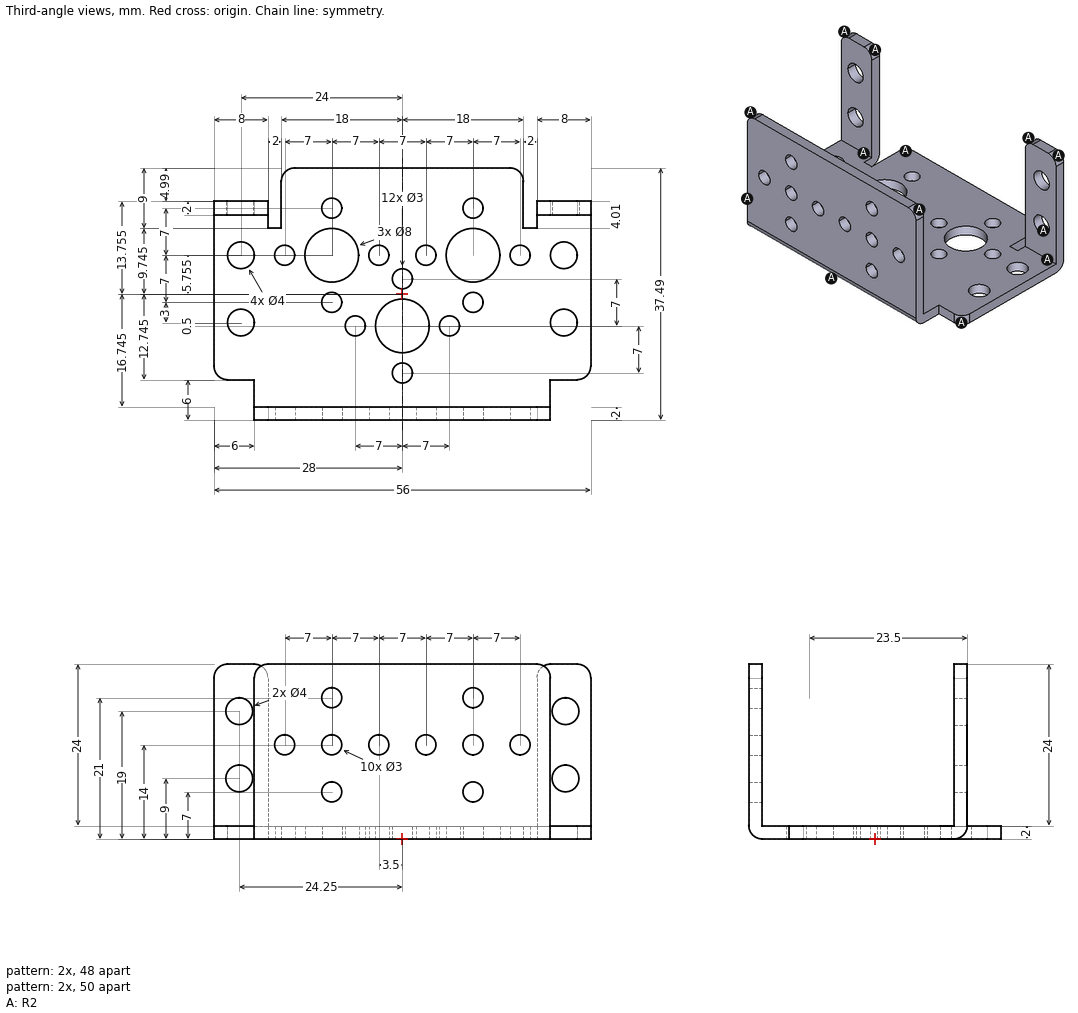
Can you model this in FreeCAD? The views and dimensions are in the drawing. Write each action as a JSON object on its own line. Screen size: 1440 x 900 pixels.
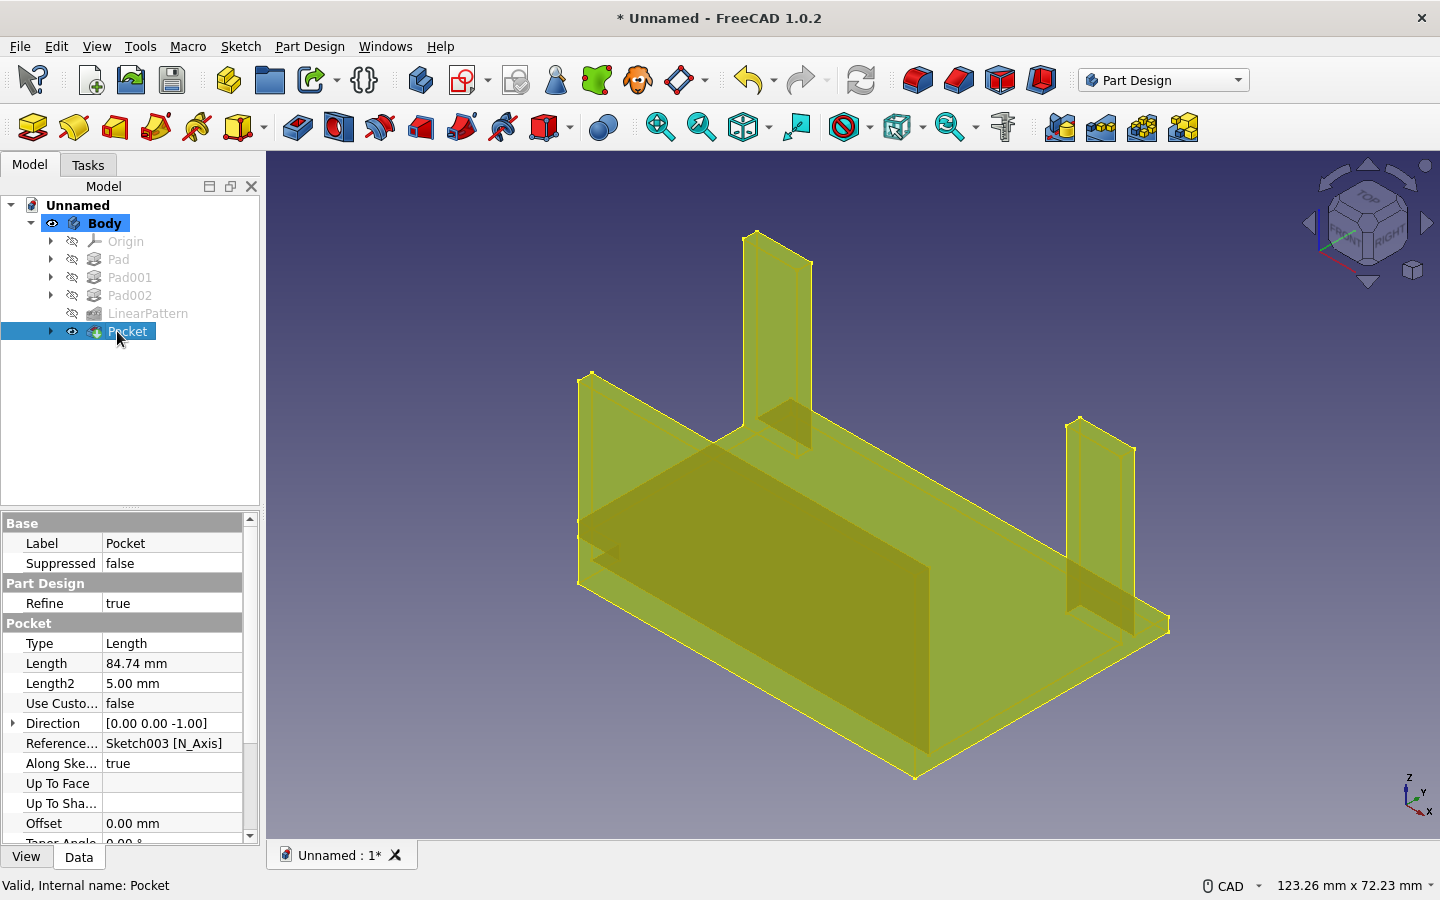
{"action": "left_click", "coordinate": [1101, 128]}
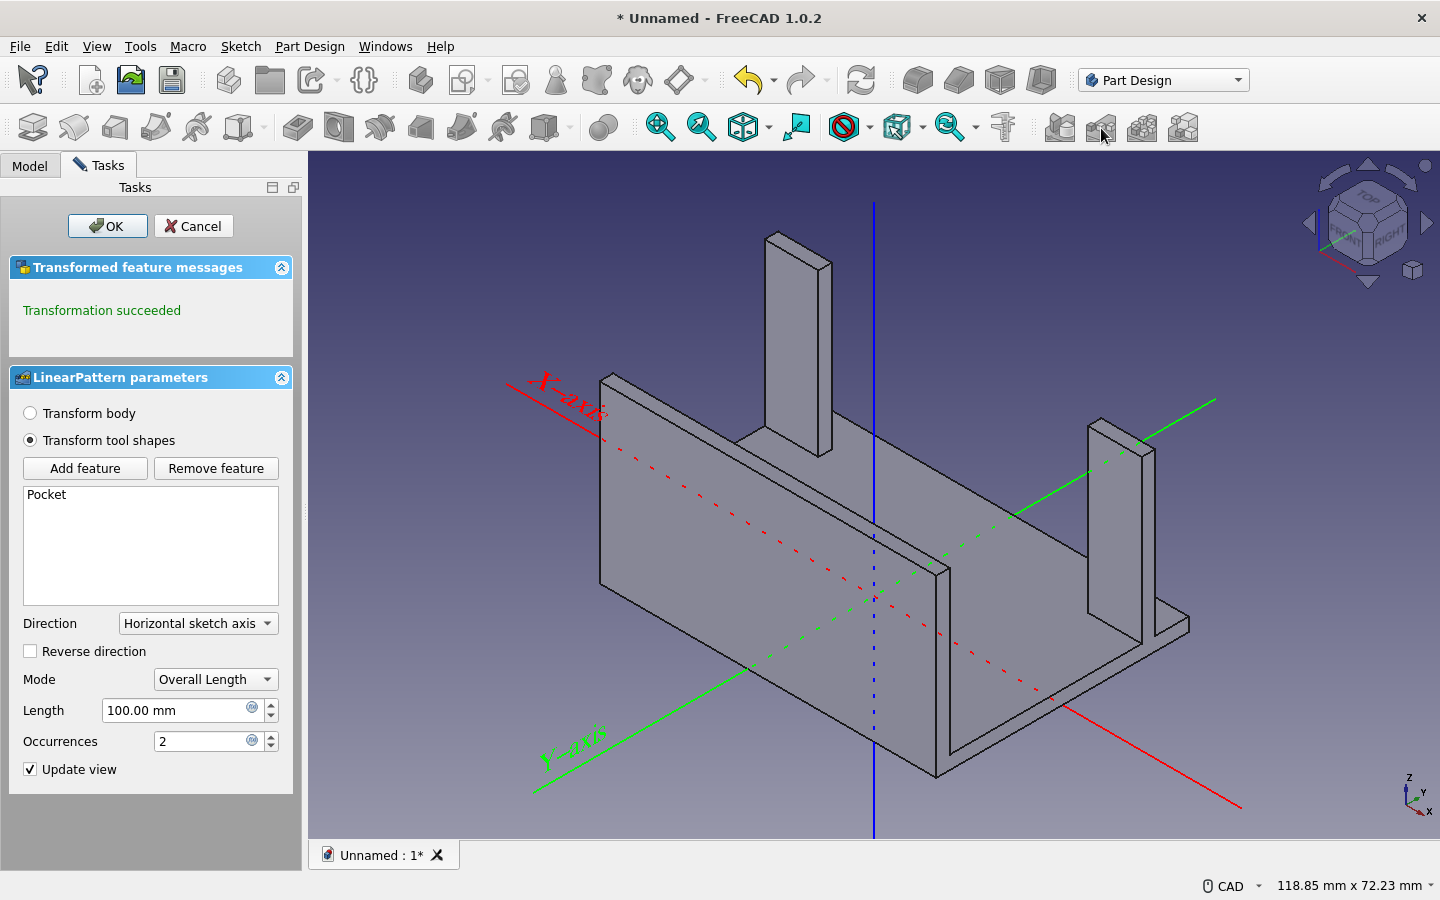
{"action": "left_click", "coordinate": [199, 624]}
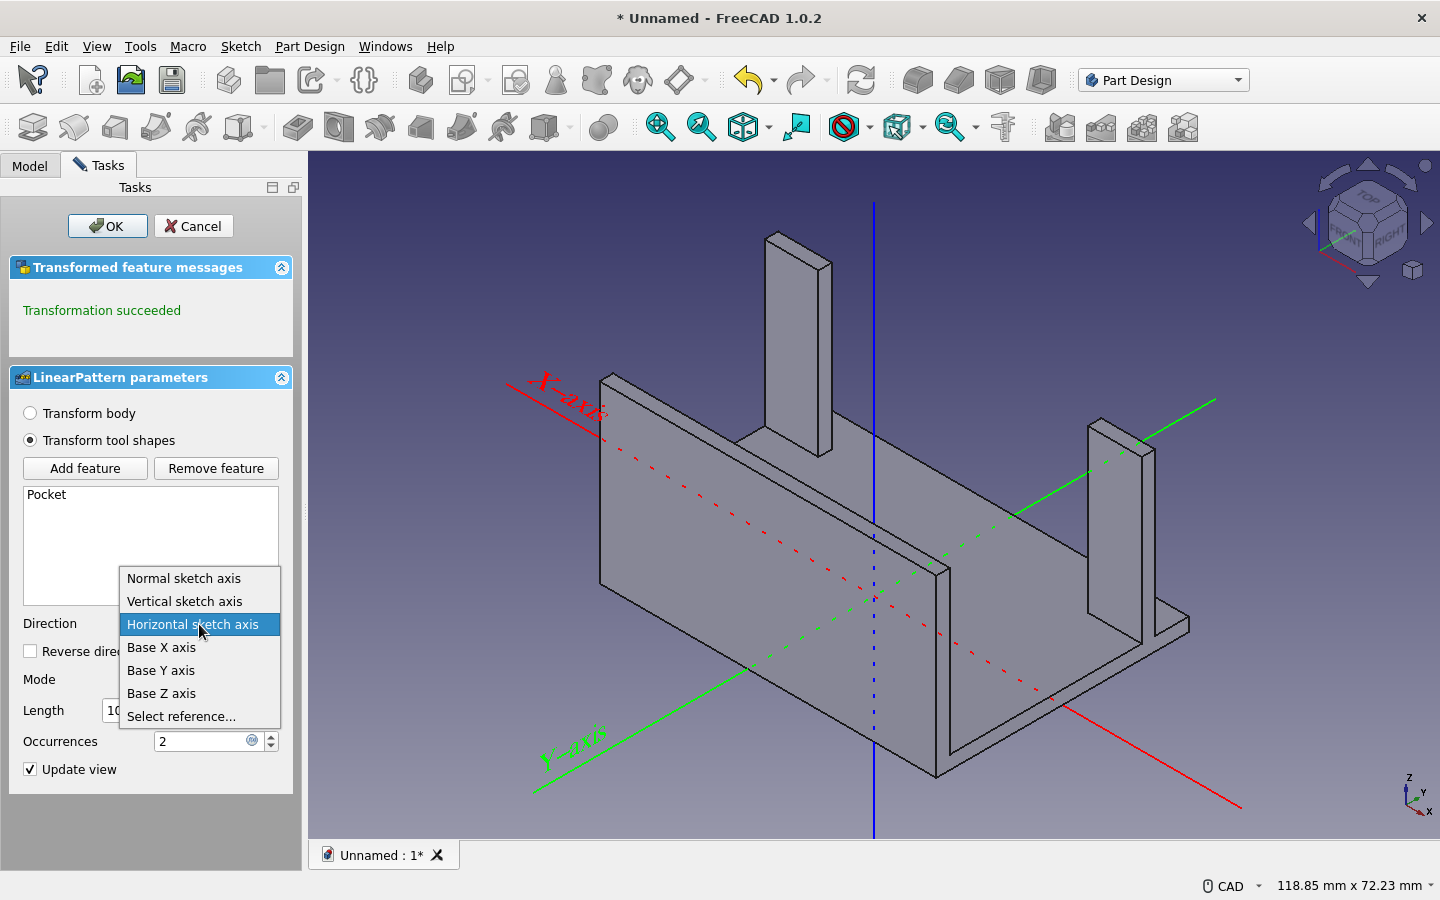
{"action": "left_click", "coordinate": [198, 648]}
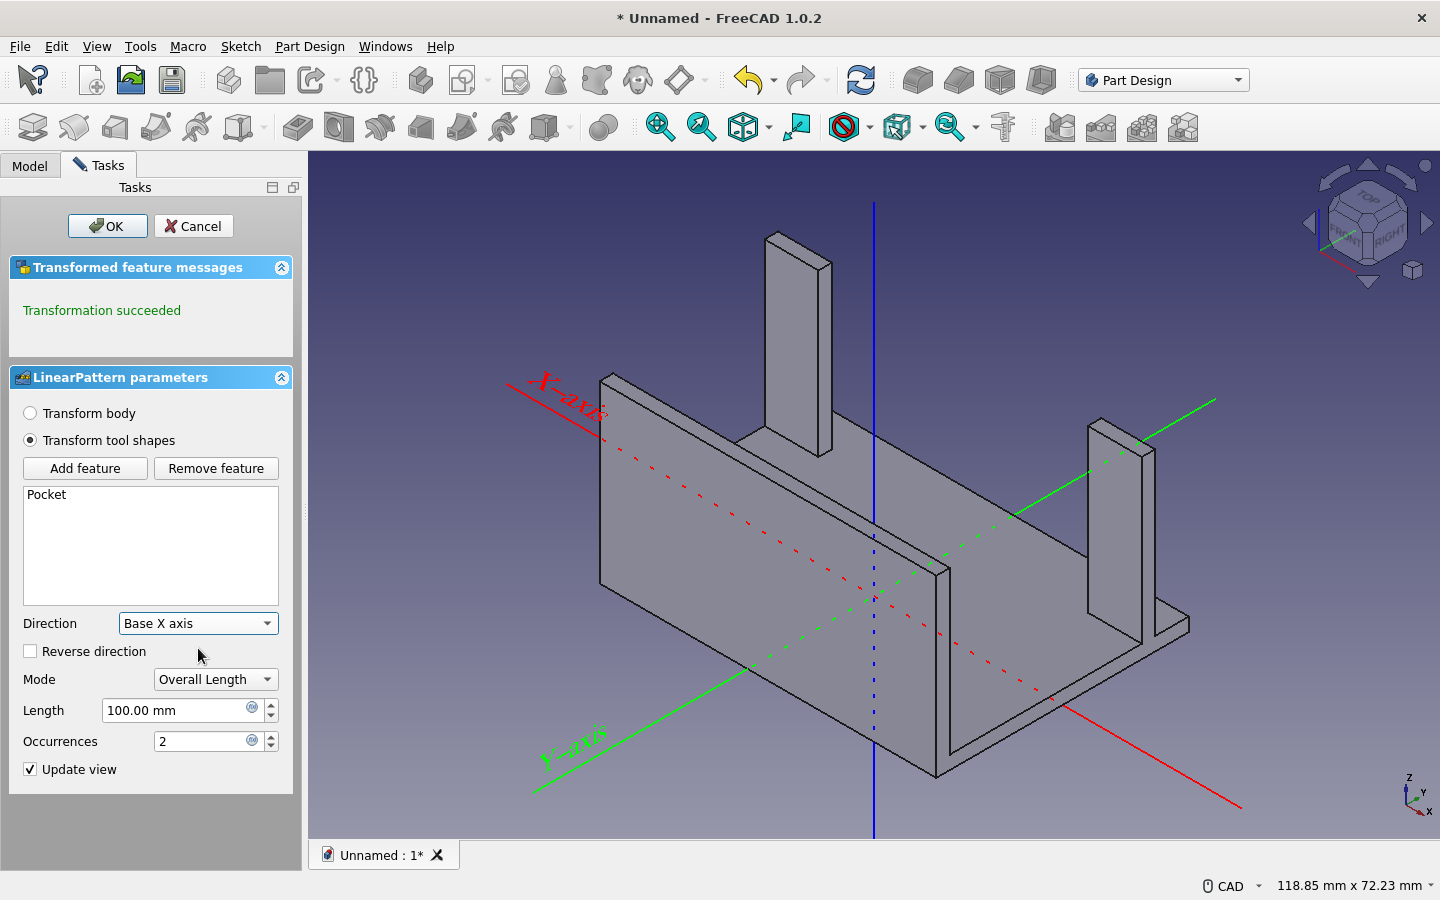
{"action": "left_click", "coordinate": [216, 680]}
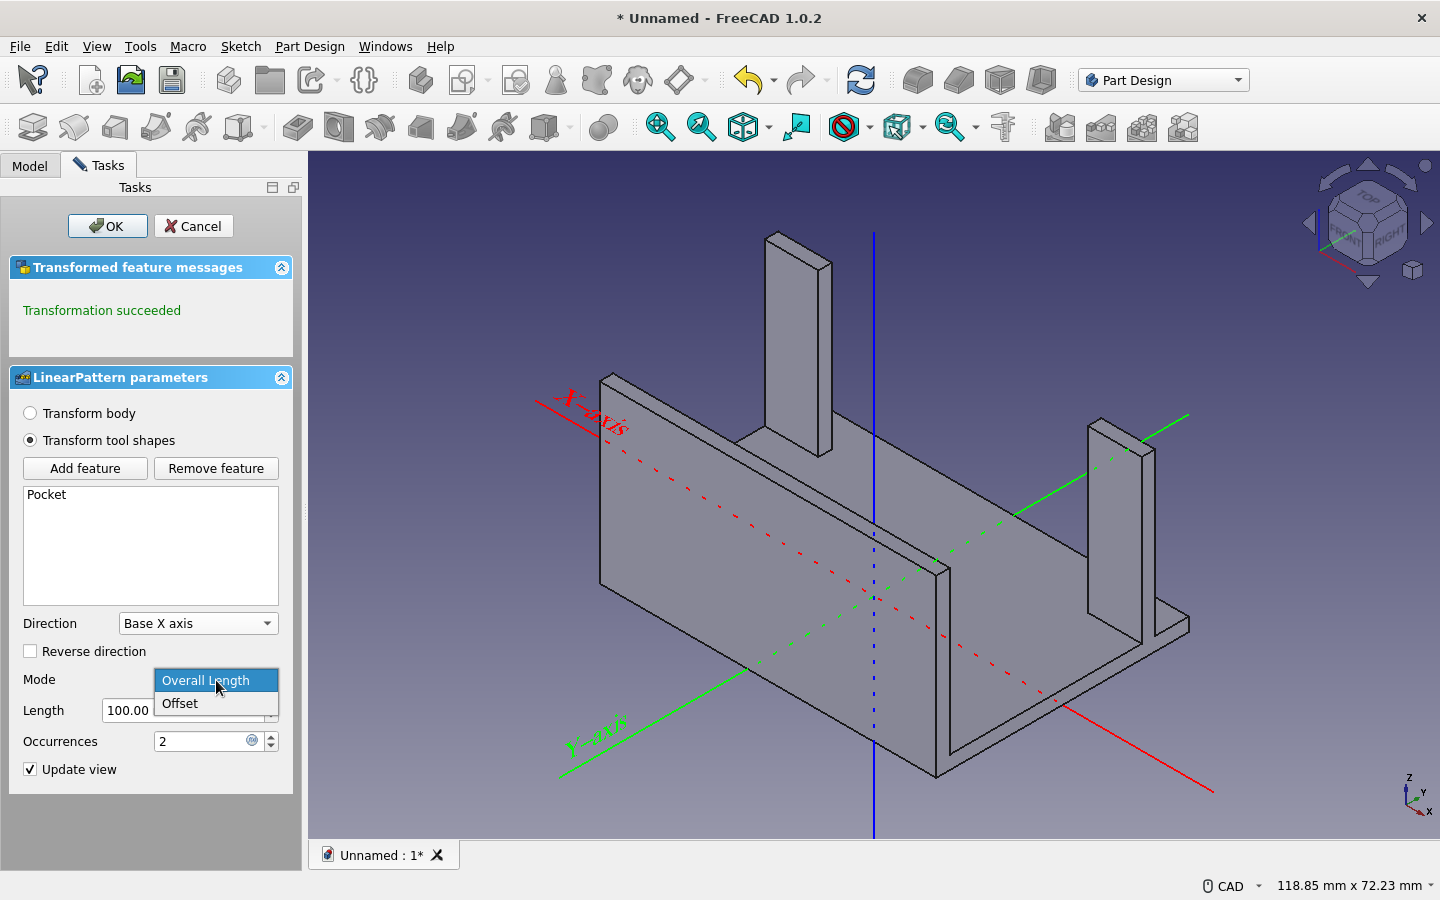
{"action": "left_click", "coordinate": [214, 704]}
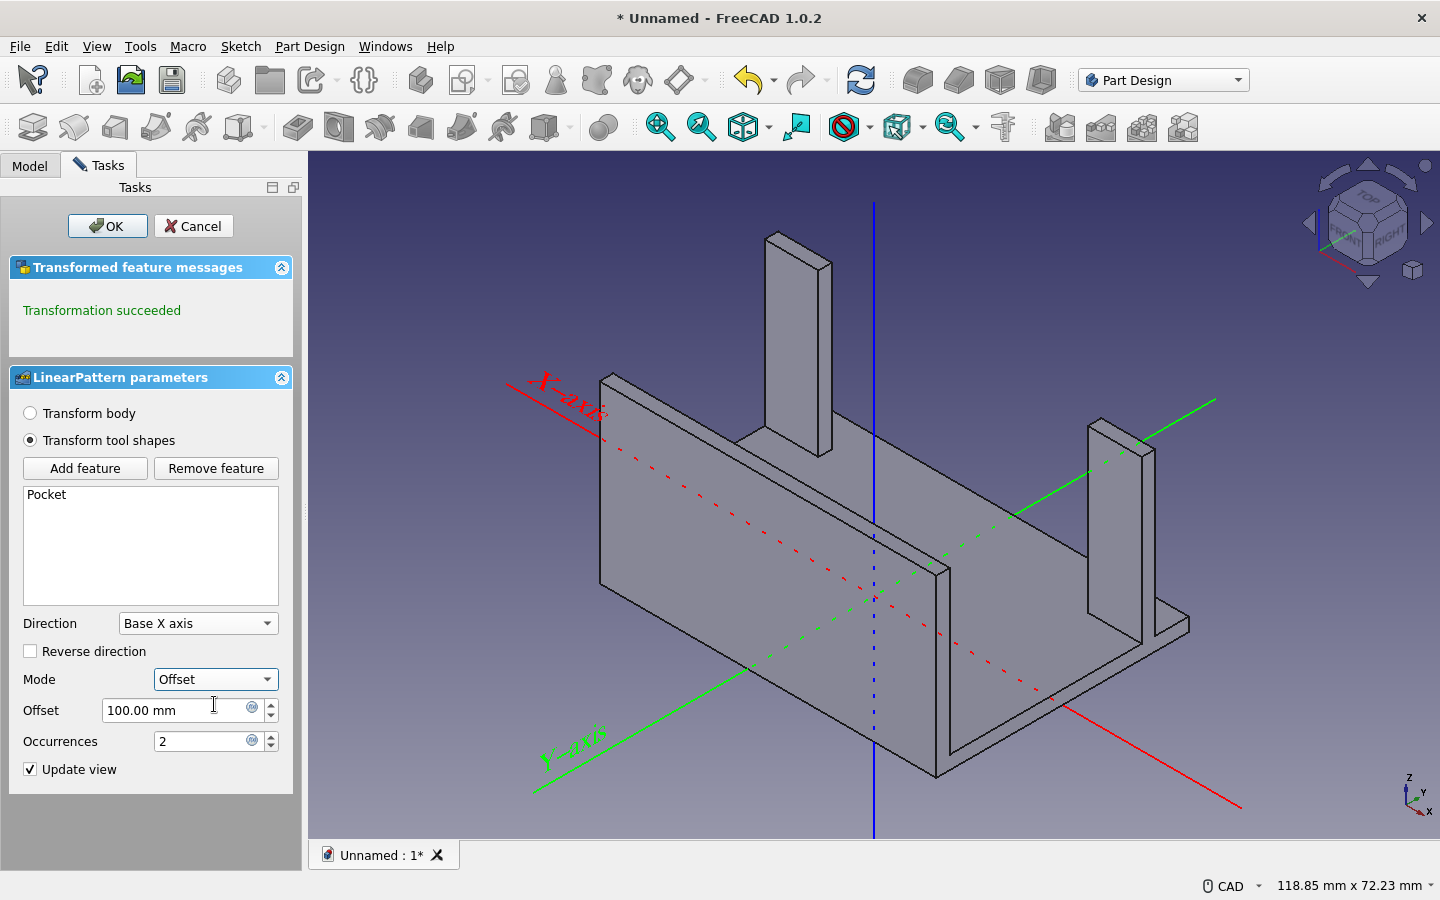
{"action": "triple_click", "coordinate": [184, 710]}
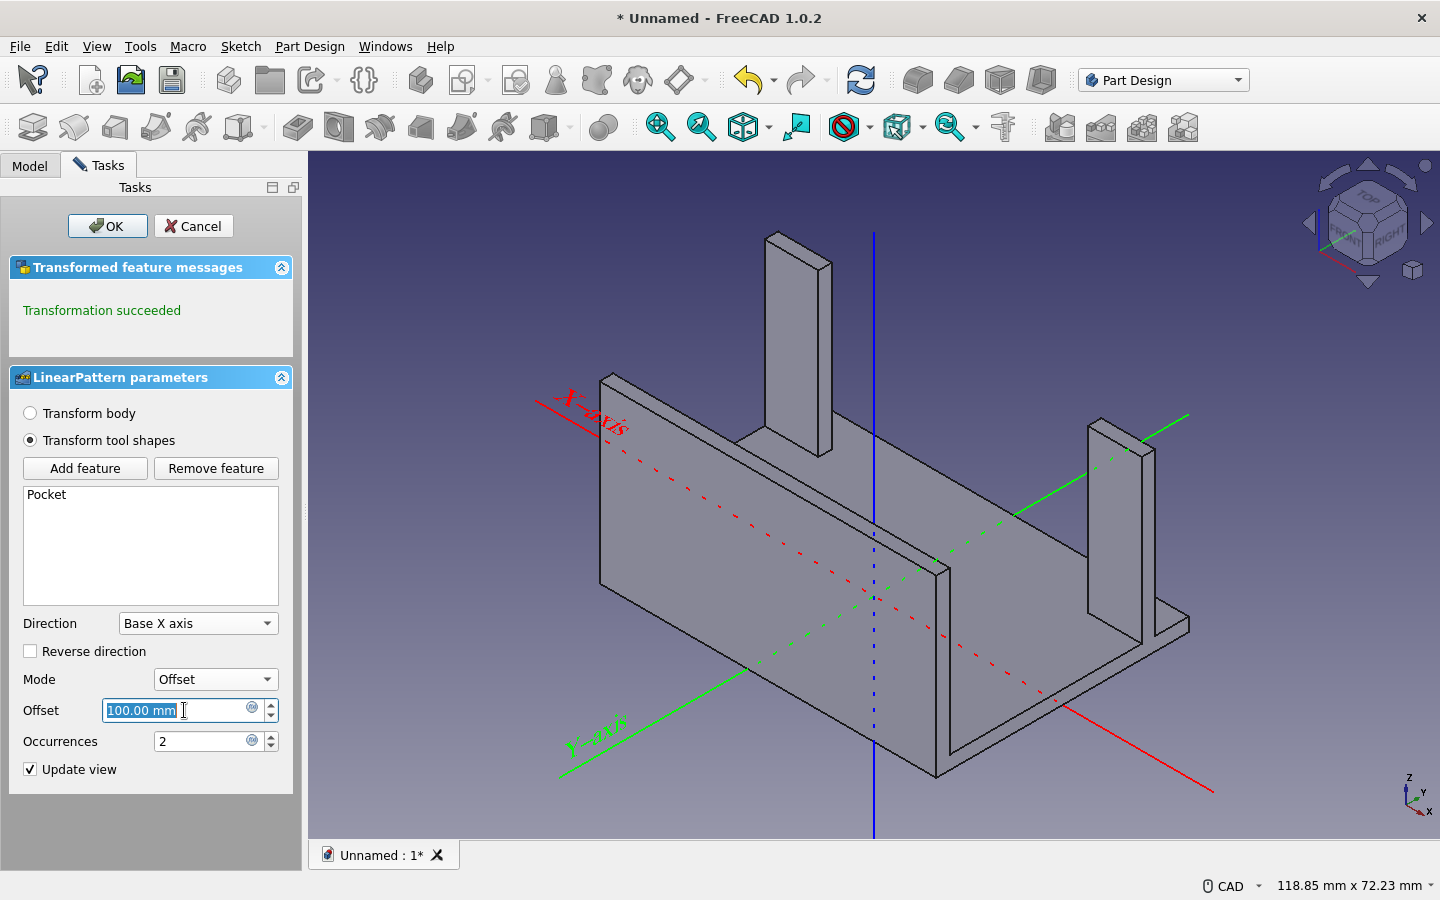
{"action": "type", "text": "50"}
{"action": "key", "text": "Tab"}